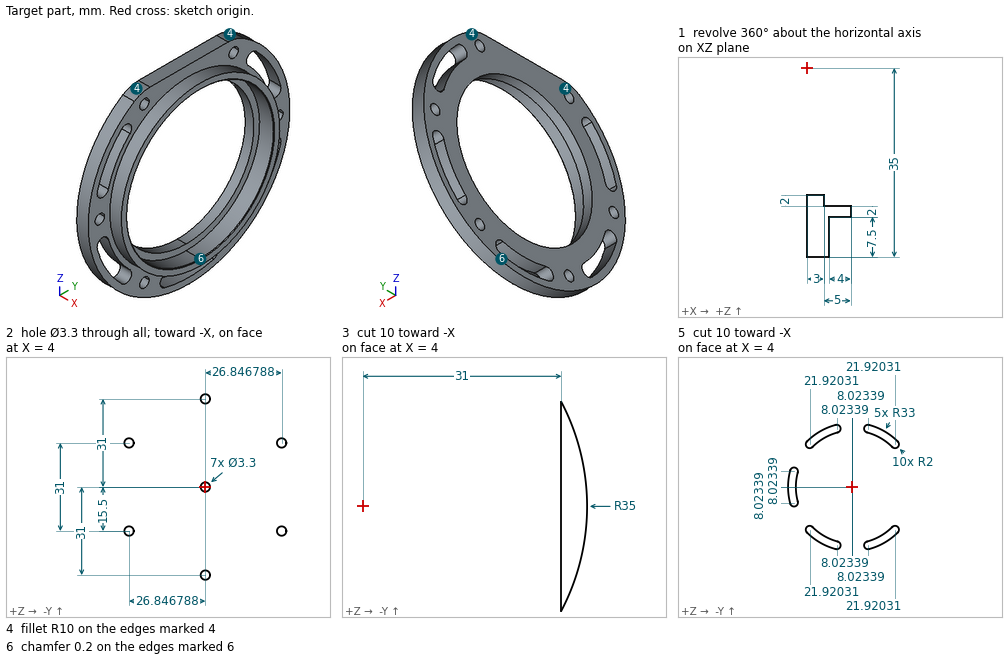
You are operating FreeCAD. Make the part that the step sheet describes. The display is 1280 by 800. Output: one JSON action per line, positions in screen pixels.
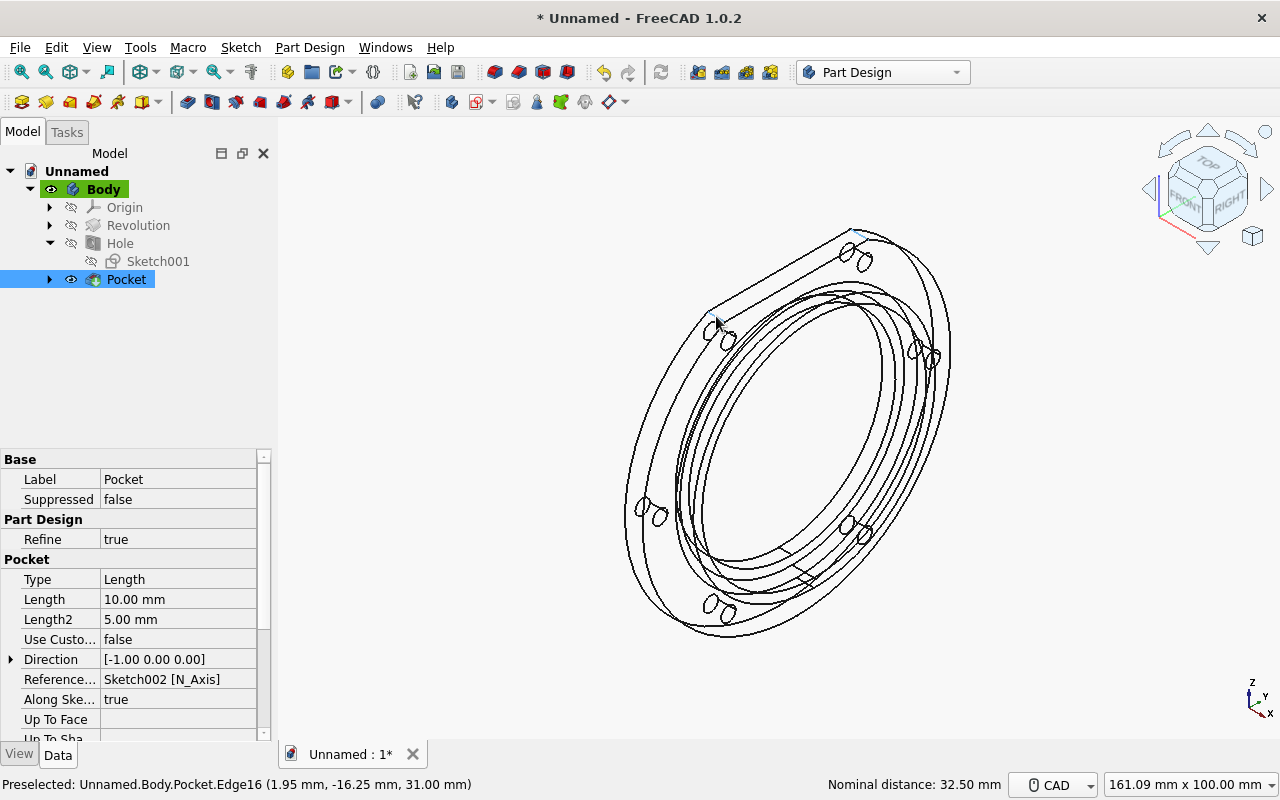
{"action": "key", "text": "v 1"}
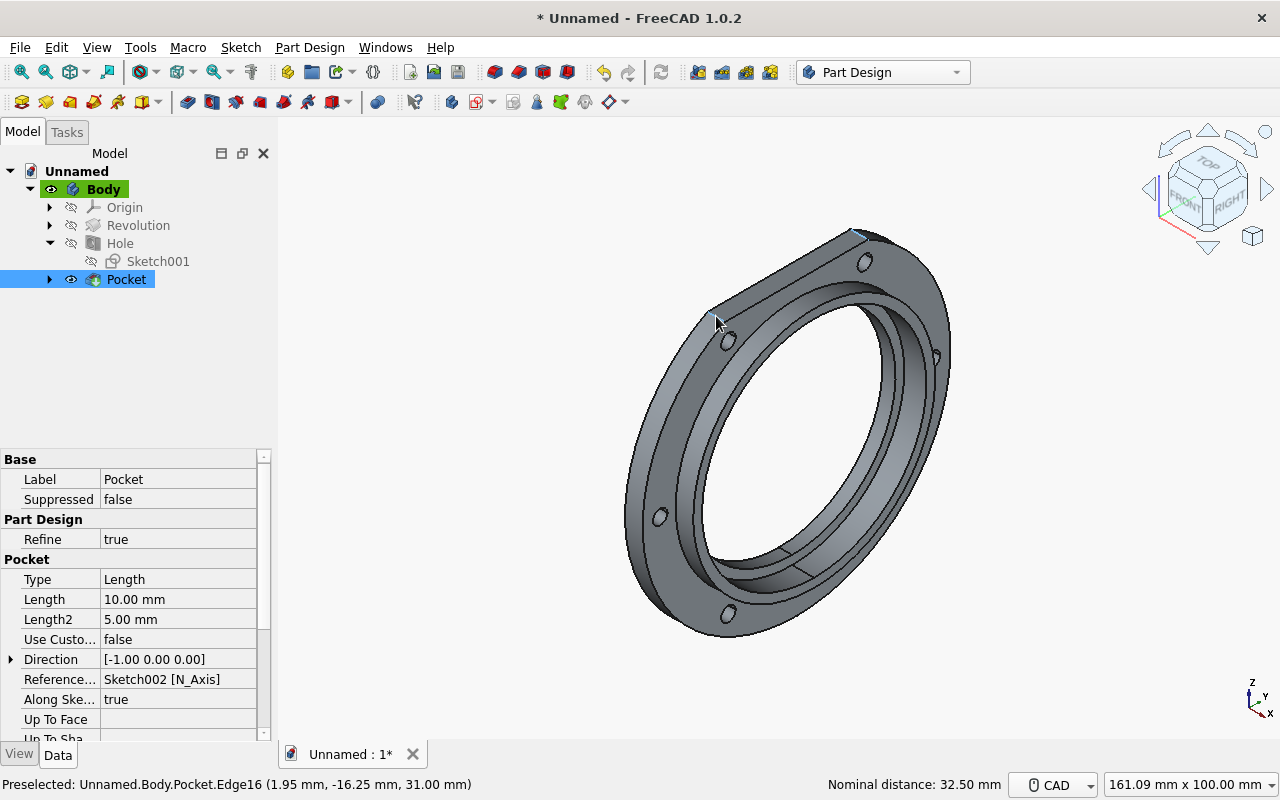
{"action": "left_click", "coordinate": [496, 72]}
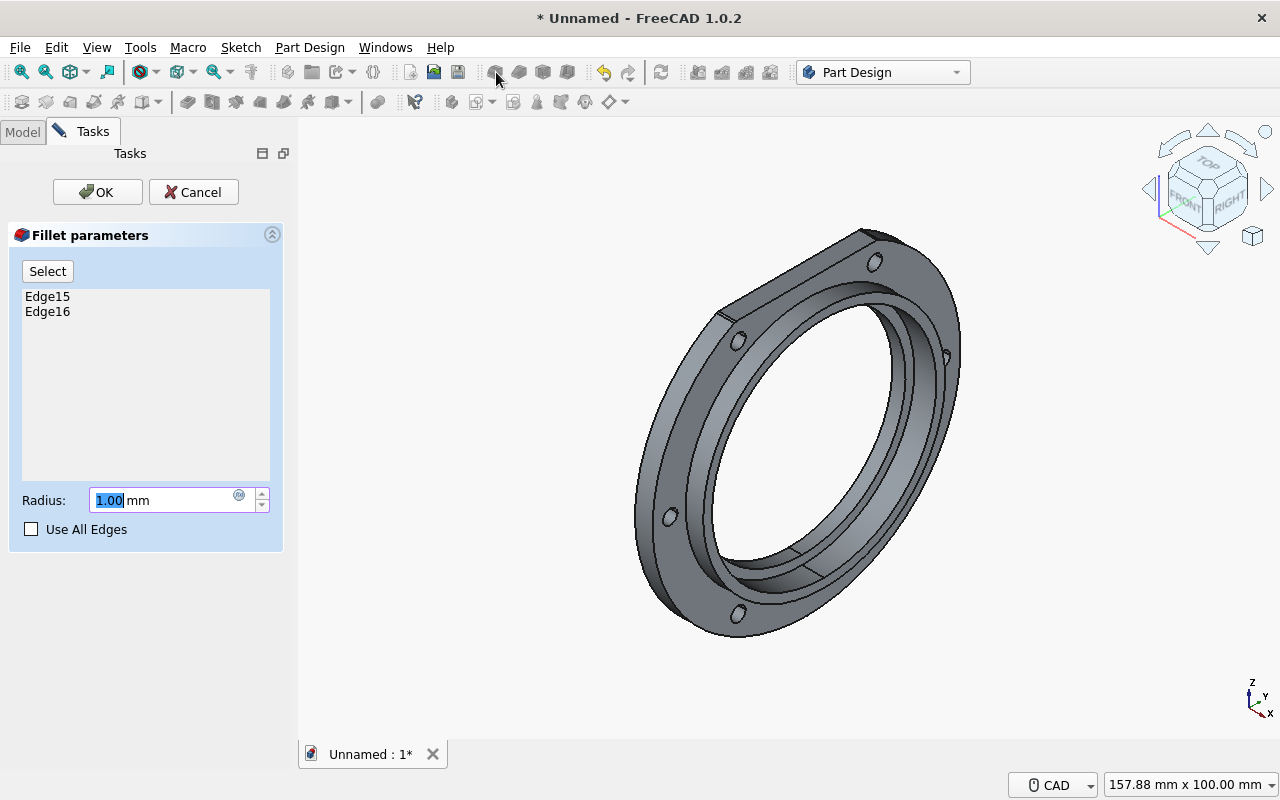
{"action": "type", "text": "10"}
{"action": "key", "text": "Tab"}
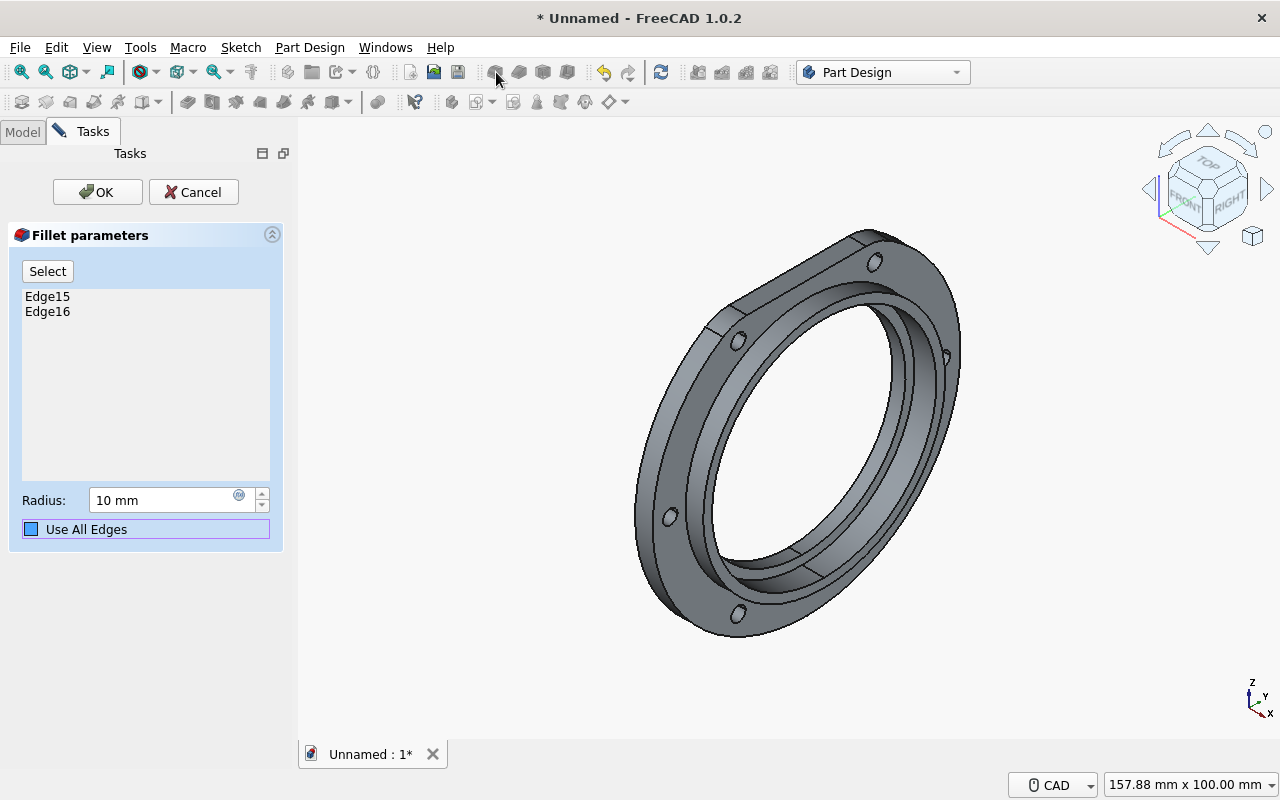
{"action": "left_click", "coordinate": [98, 192]}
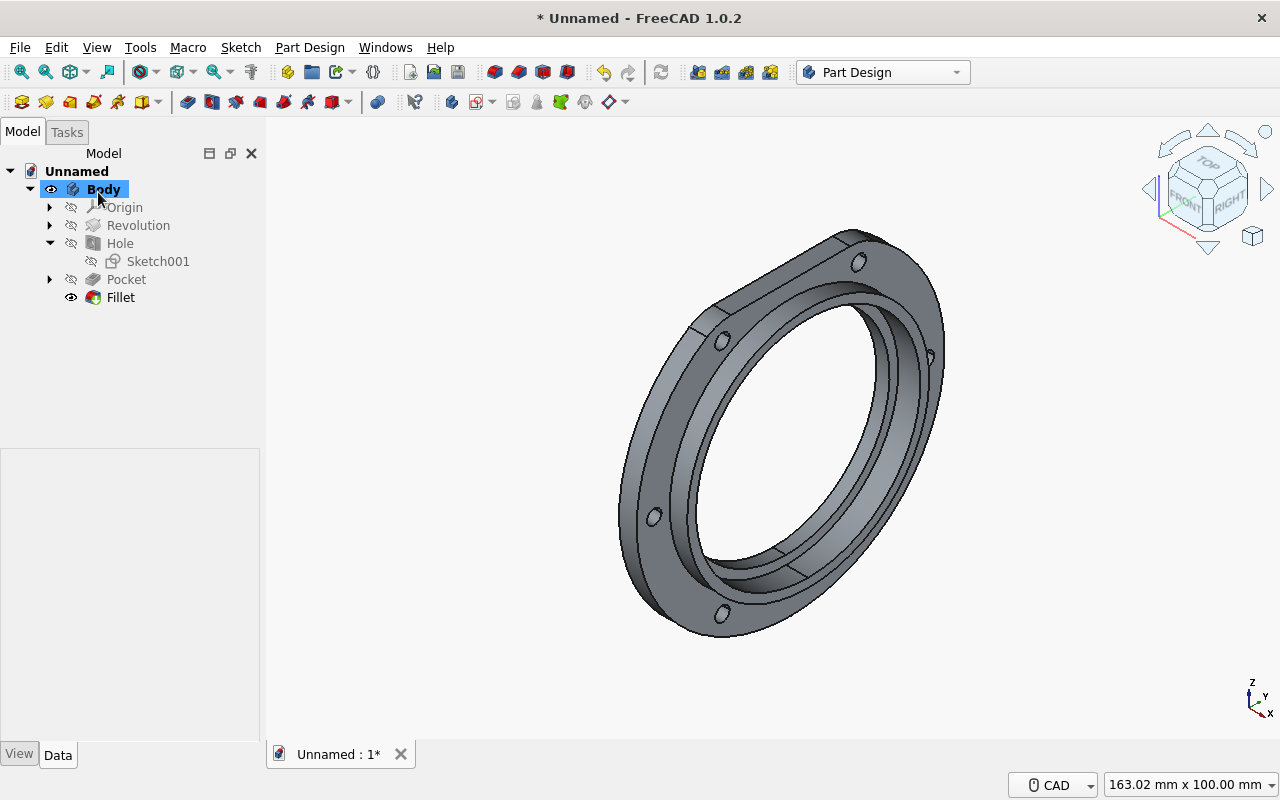
{"action": "left_click", "coordinate": [659, 476]}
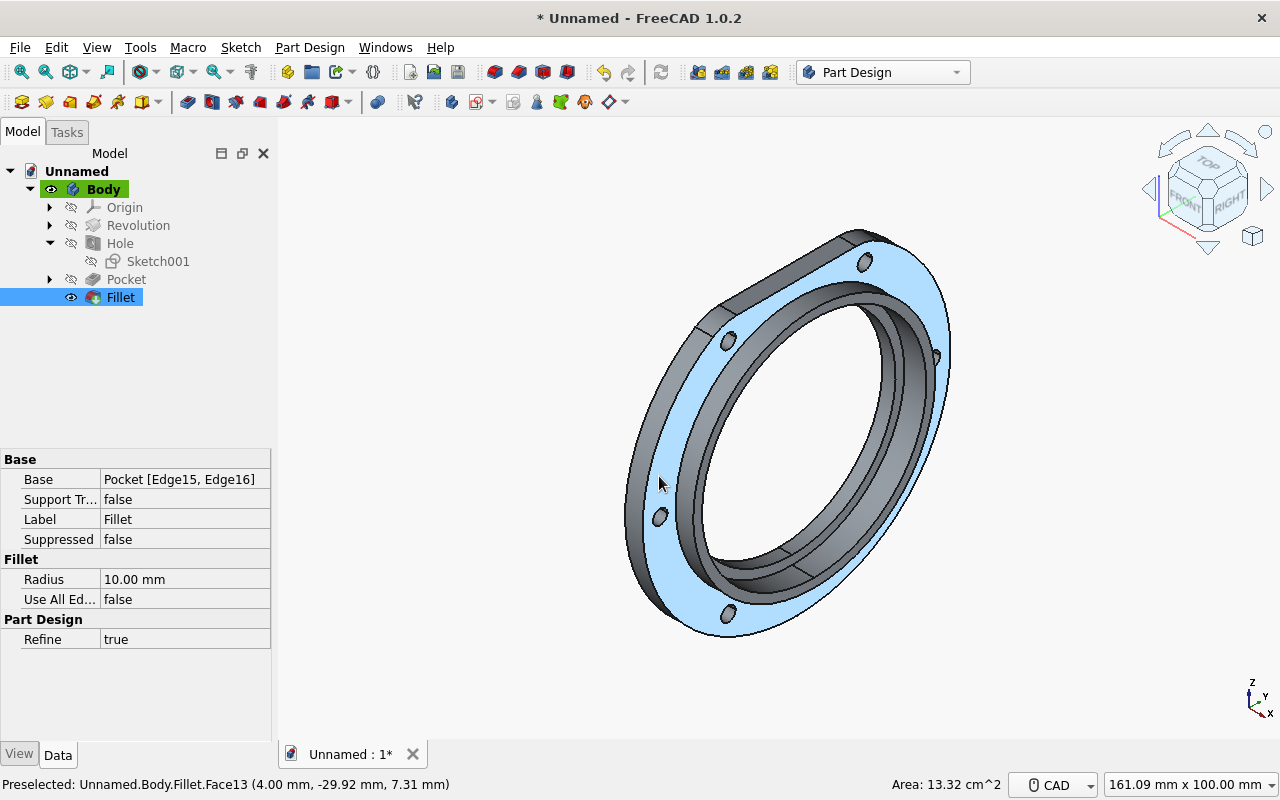
{"action": "left_click", "coordinate": [476, 102]}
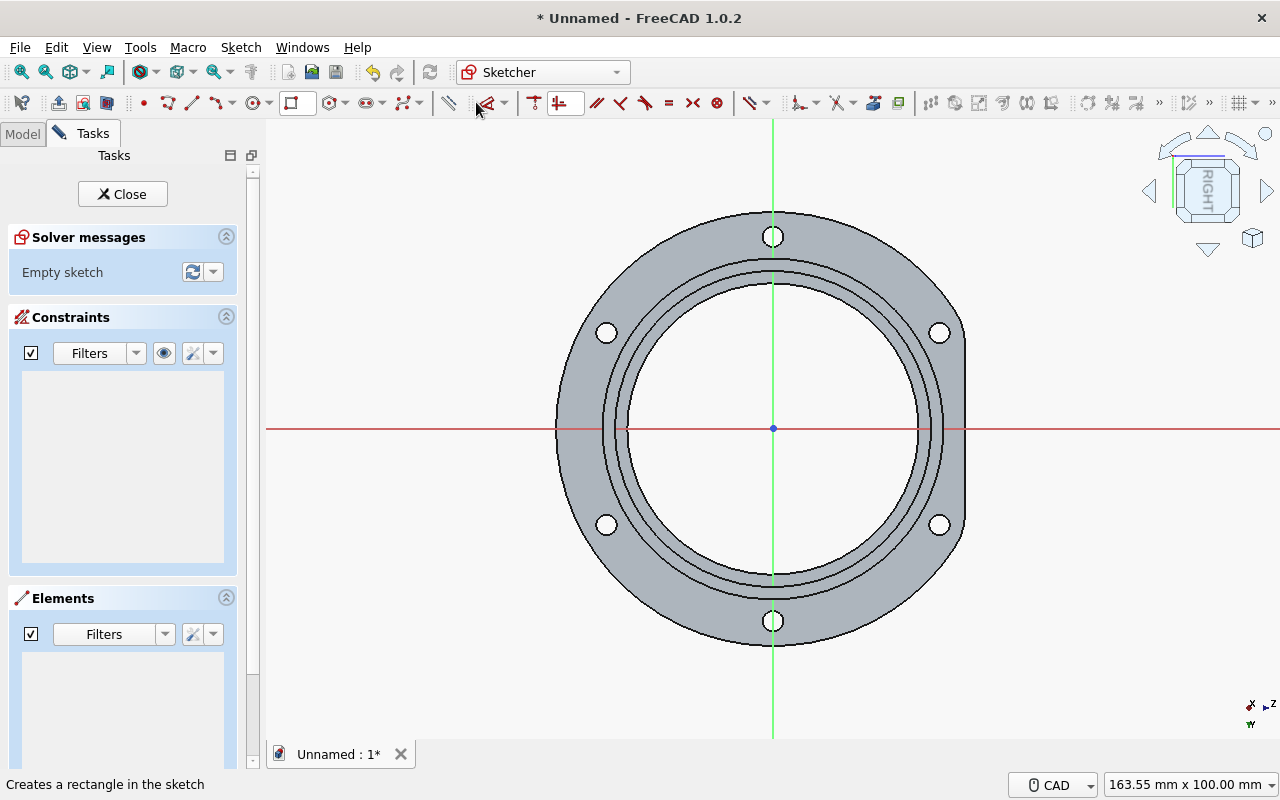
{"action": "left_click", "coordinate": [108, 104]}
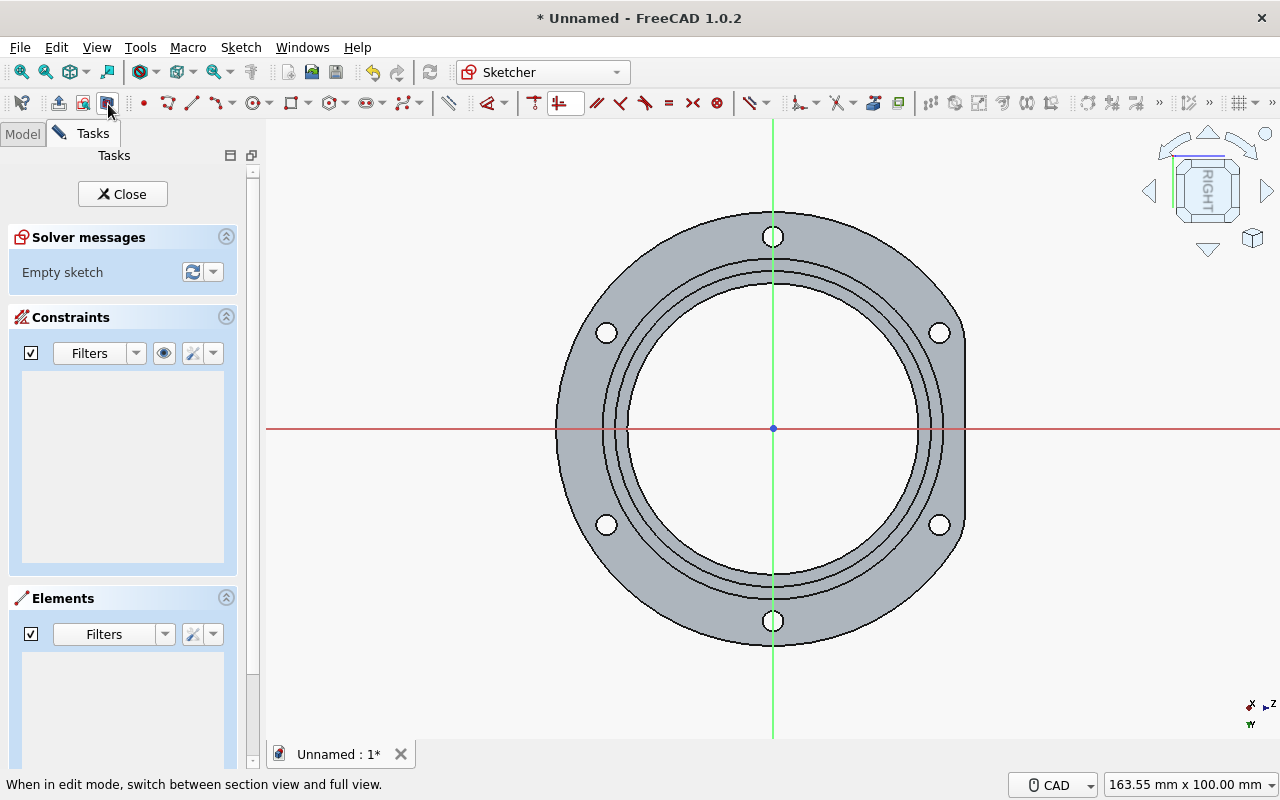
{"action": "left_click", "coordinate": [216, 104]}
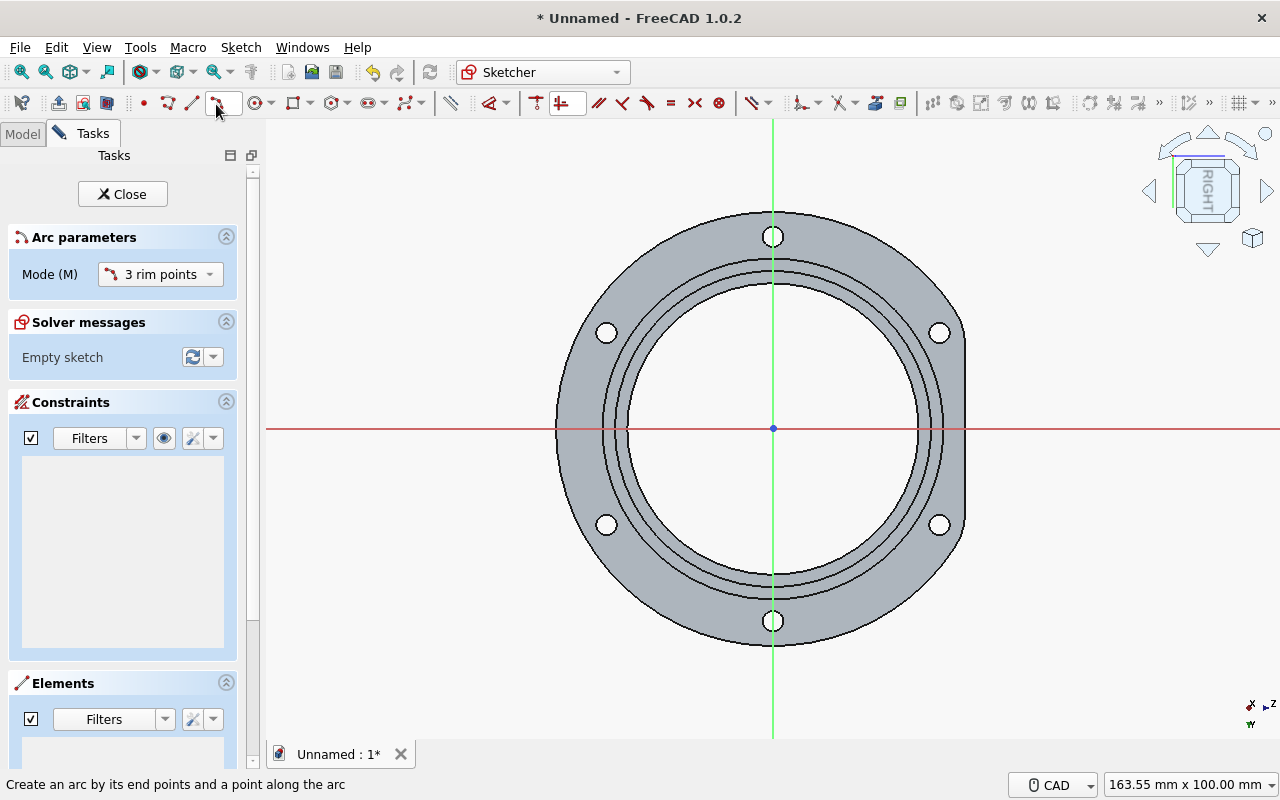
{"action": "left_click", "coordinate": [646, 556]}
{"action": "left_click", "coordinate": [628, 574]}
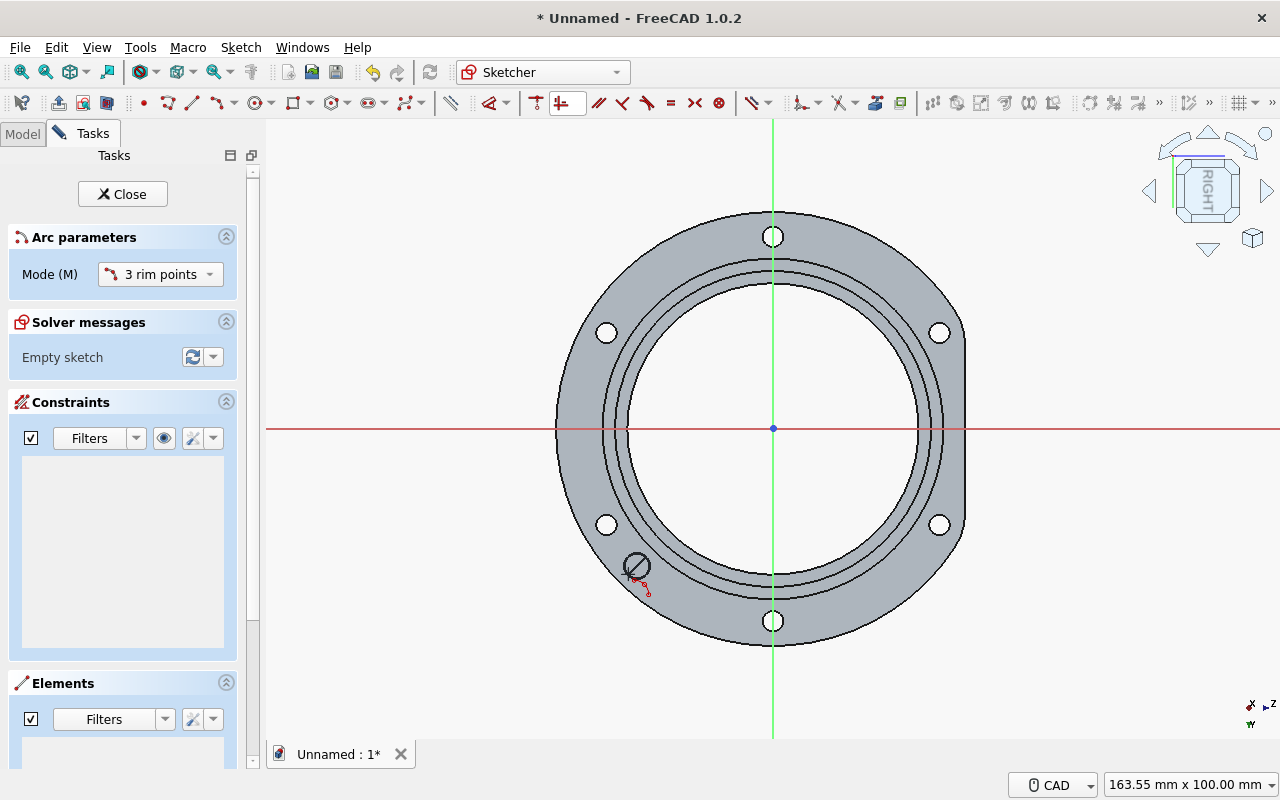
{"action": "scroll", "coordinate": [628, 556], "scroll_direction": "up", "scroll_amount": 2}